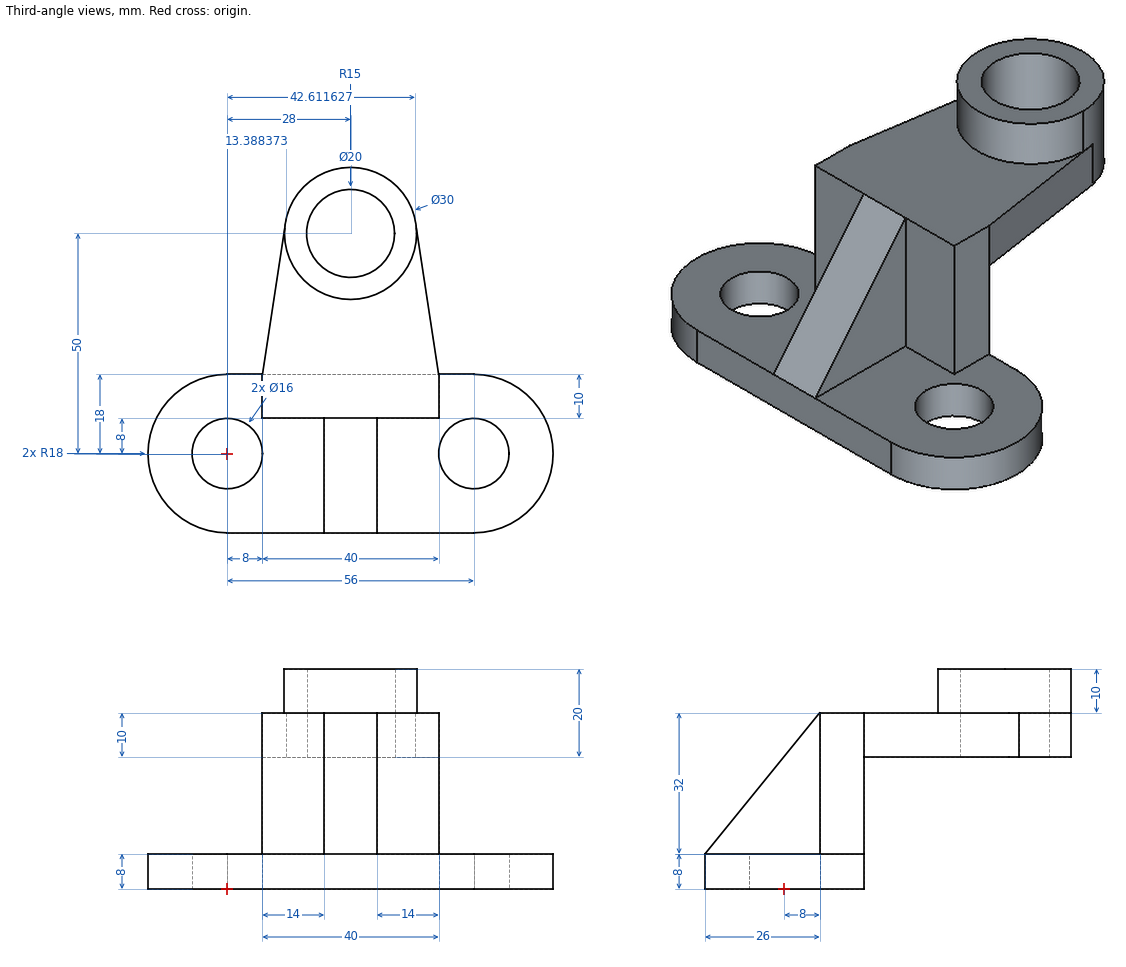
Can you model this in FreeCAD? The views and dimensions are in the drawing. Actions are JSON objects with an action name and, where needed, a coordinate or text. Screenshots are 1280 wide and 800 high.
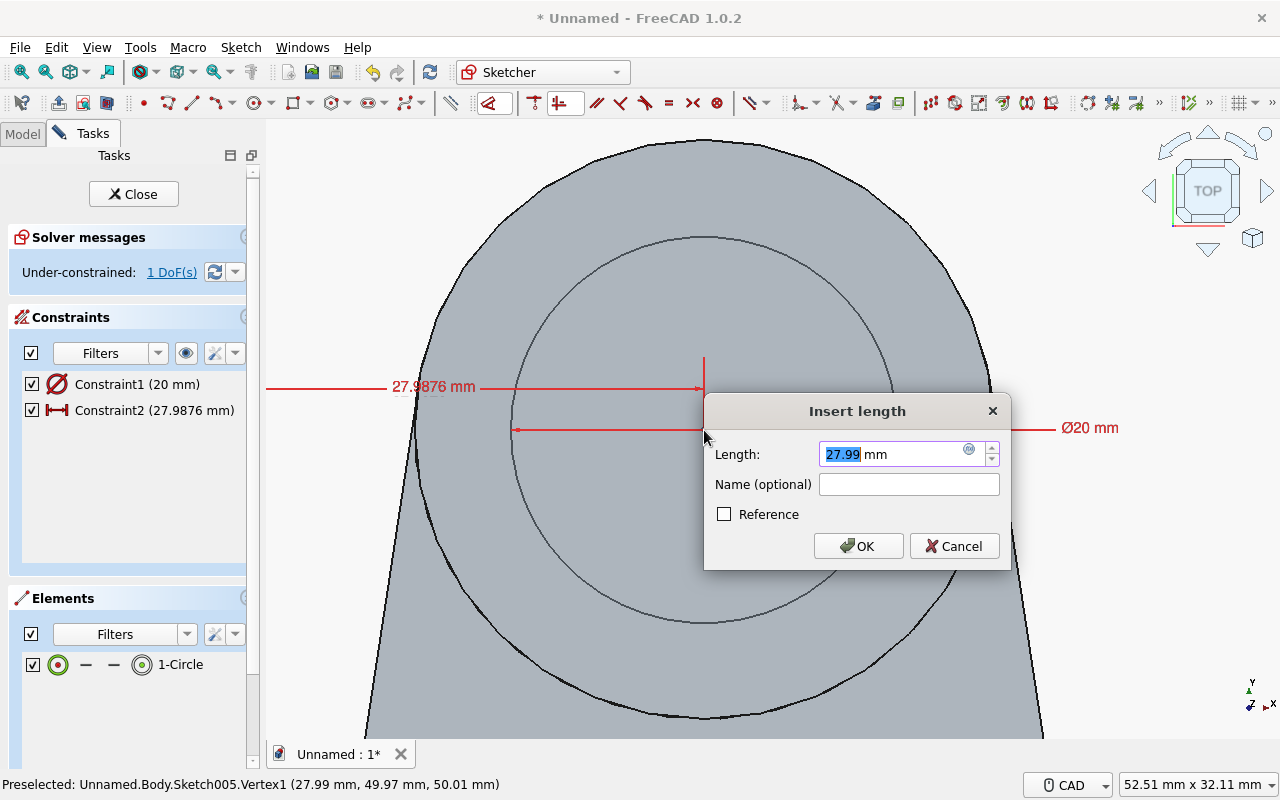
{"action": "type", "text": "28"}
{"action": "key", "text": "Return"}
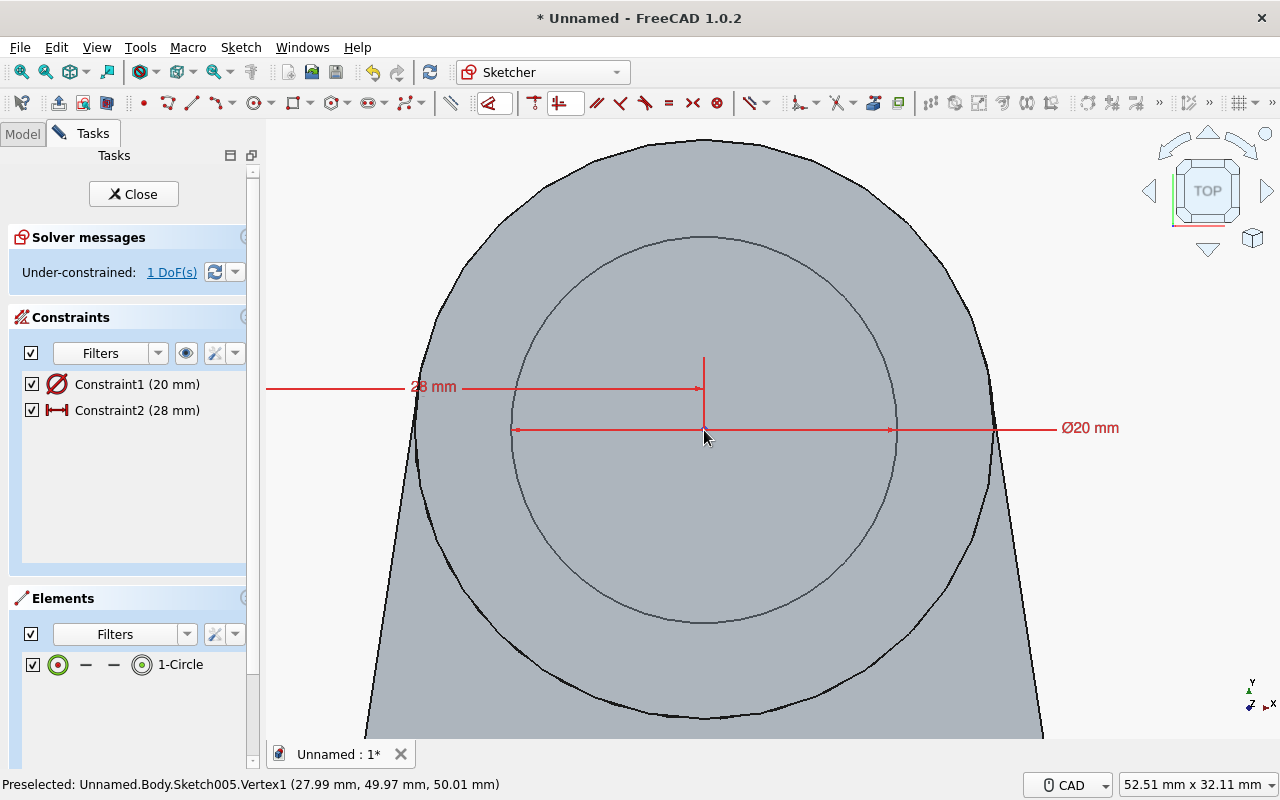
{"action": "left_click", "coordinate": [704, 430]}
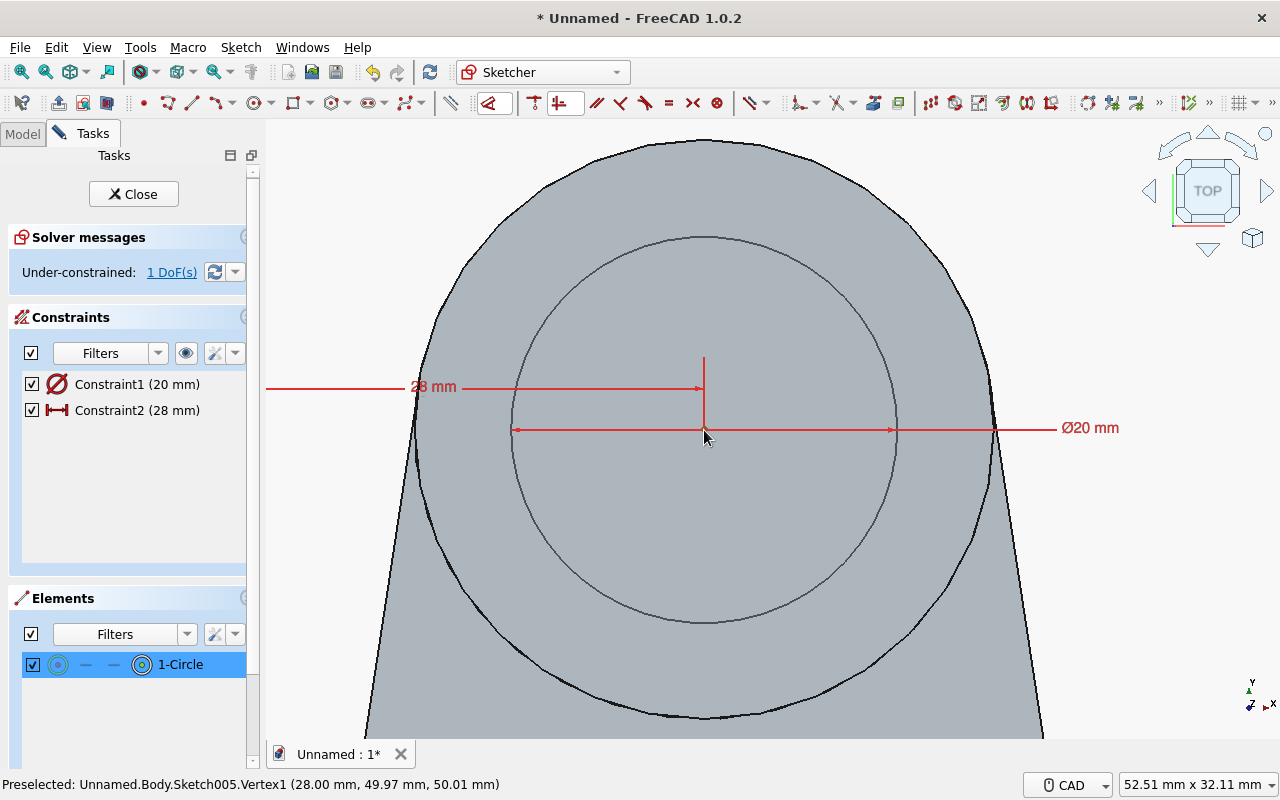
{"action": "key", "text": "i"}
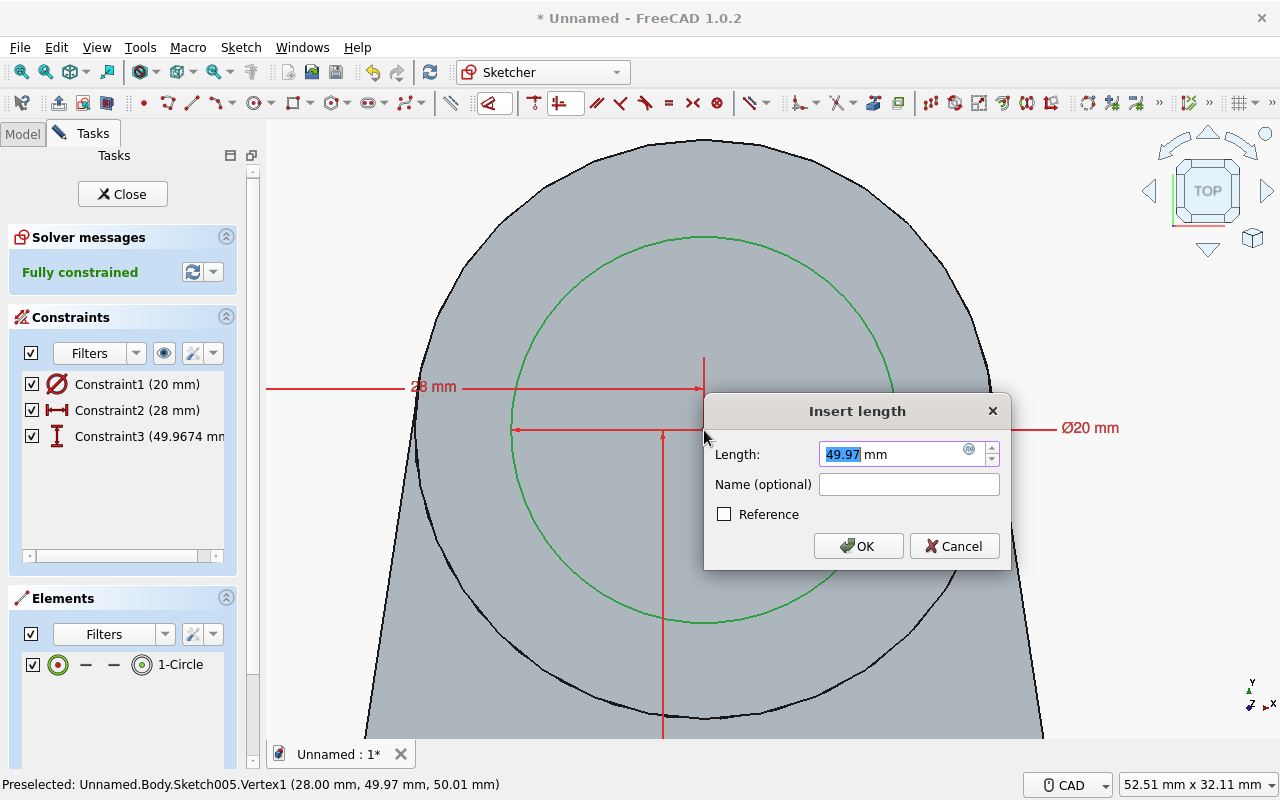
{"action": "type", "text": "50"}
{"action": "key", "text": "Return"}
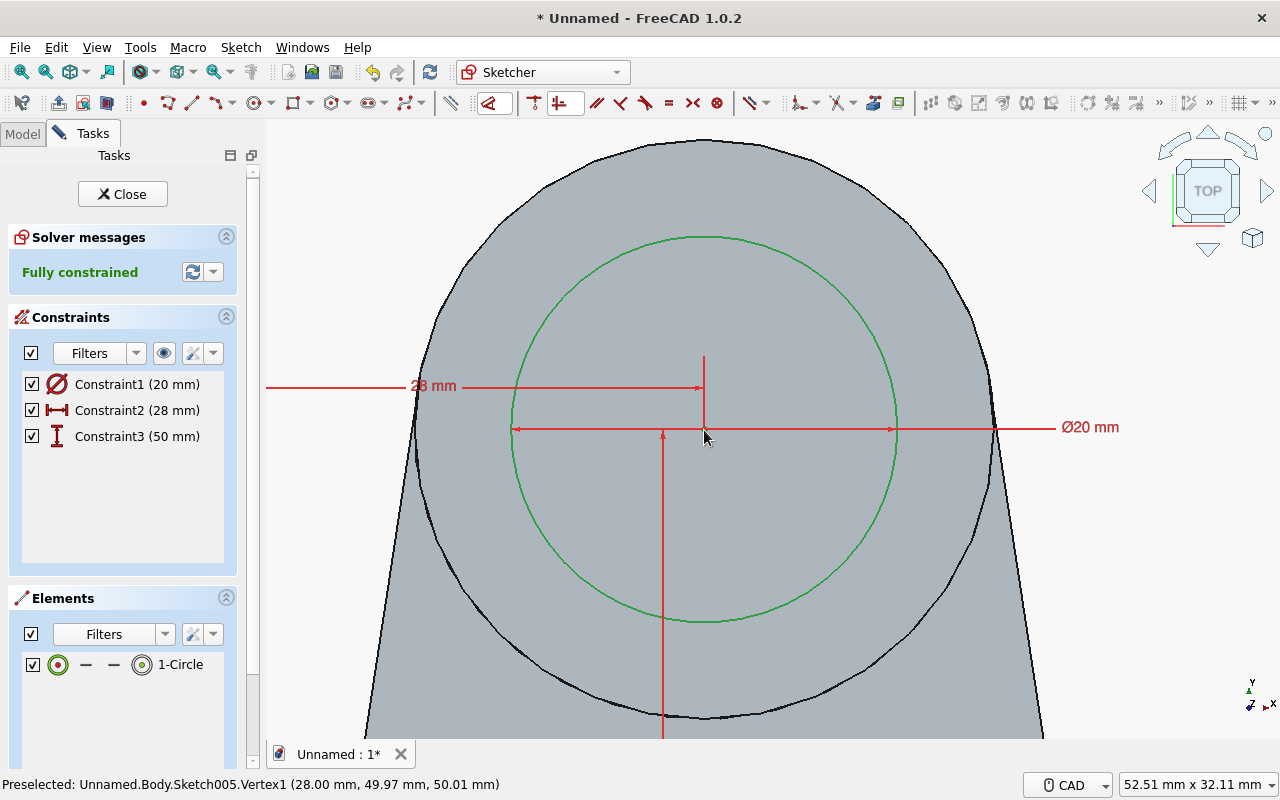
{"action": "left_click", "coordinate": [123, 194]}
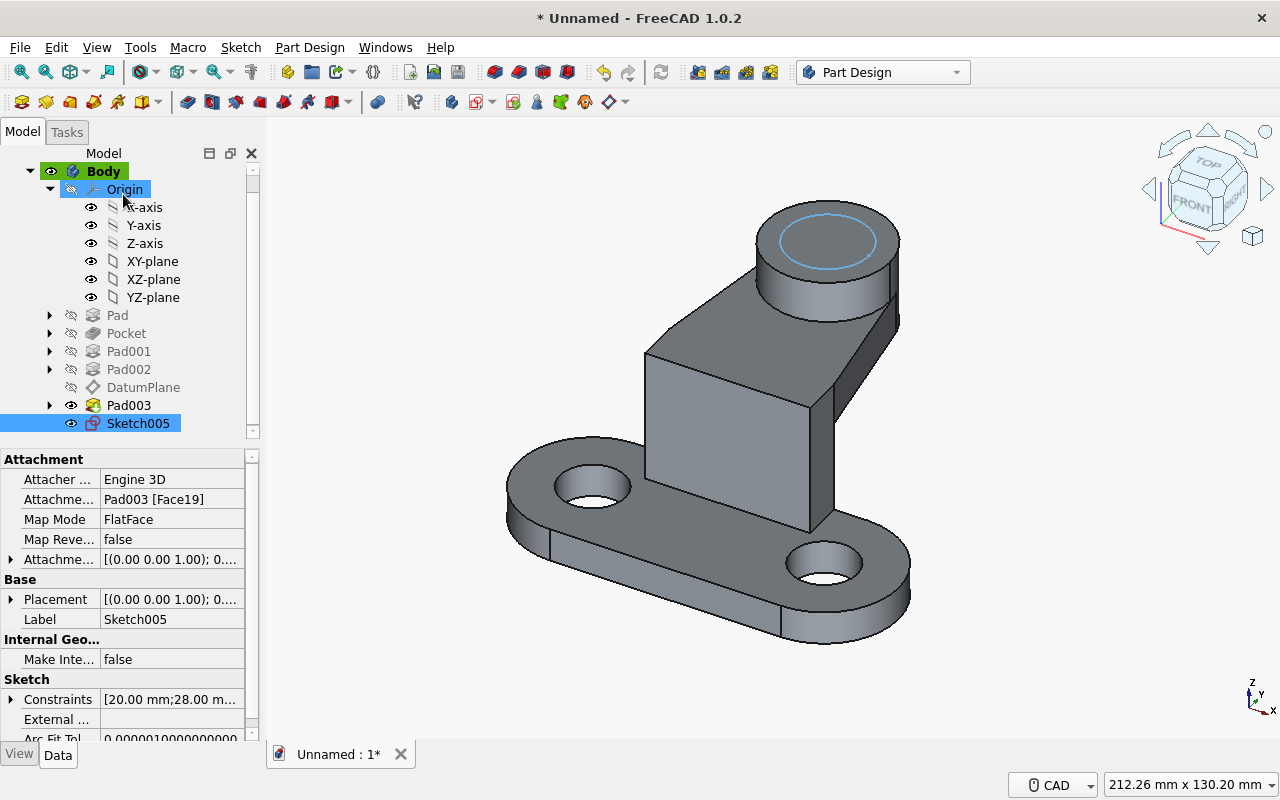
{"action": "left_click", "coordinate": [188, 102]}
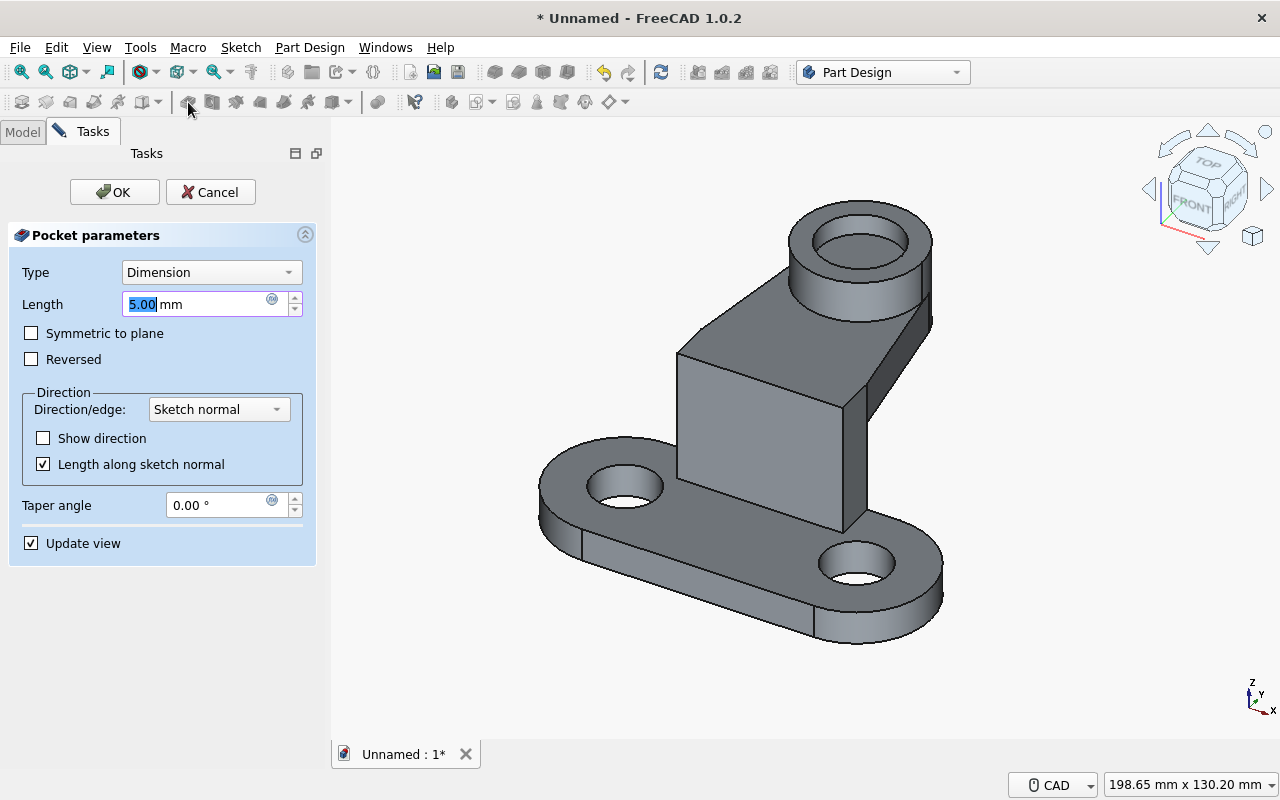
{"action": "type", "text": "20"}
{"action": "key", "text": "Tab"}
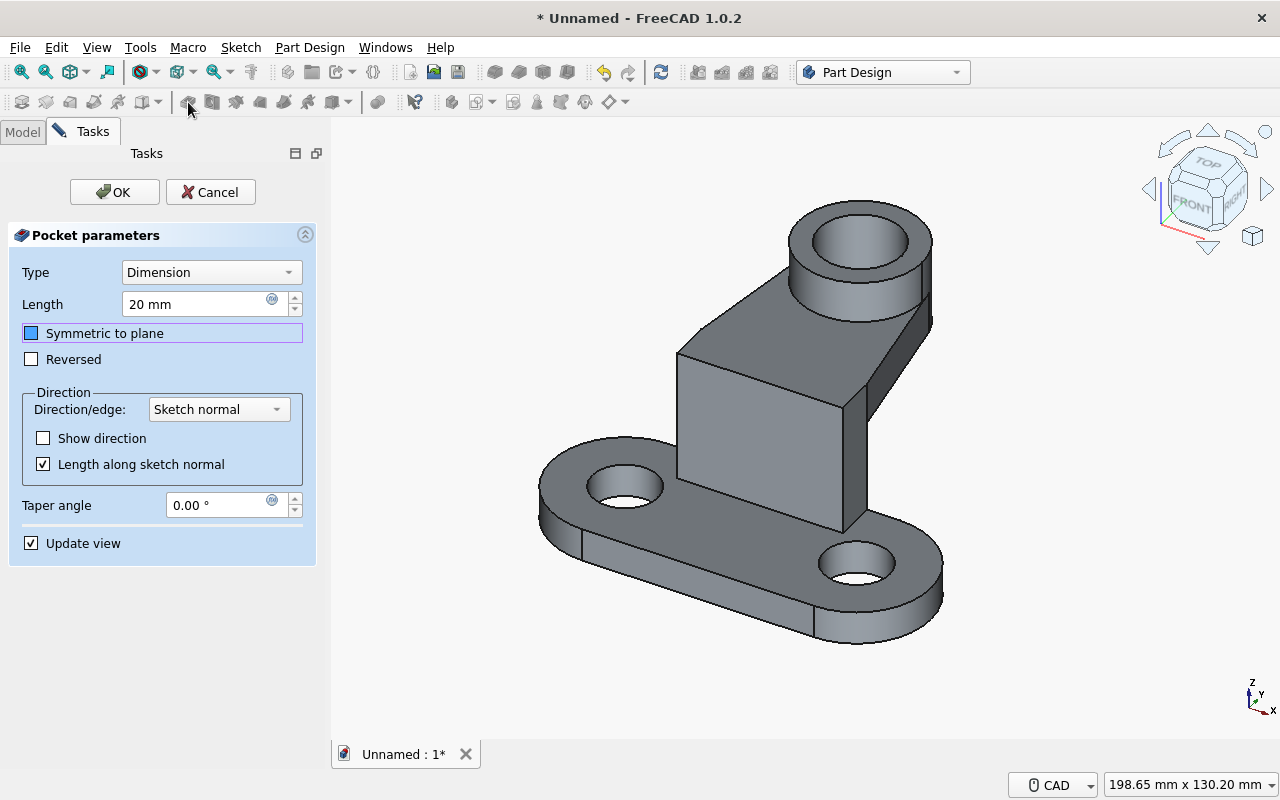
{"action": "left_click", "coordinate": [115, 192]}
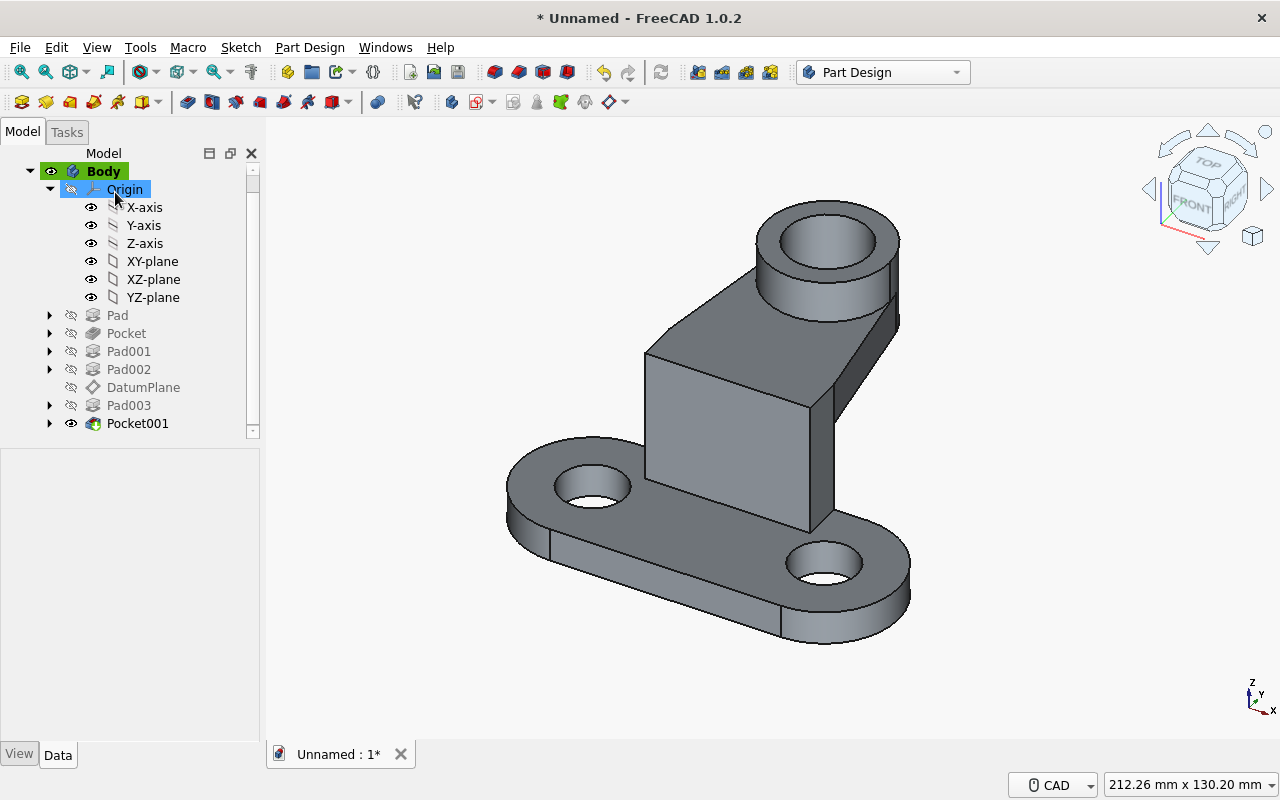
{"action": "left_click", "coordinate": [822, 422]}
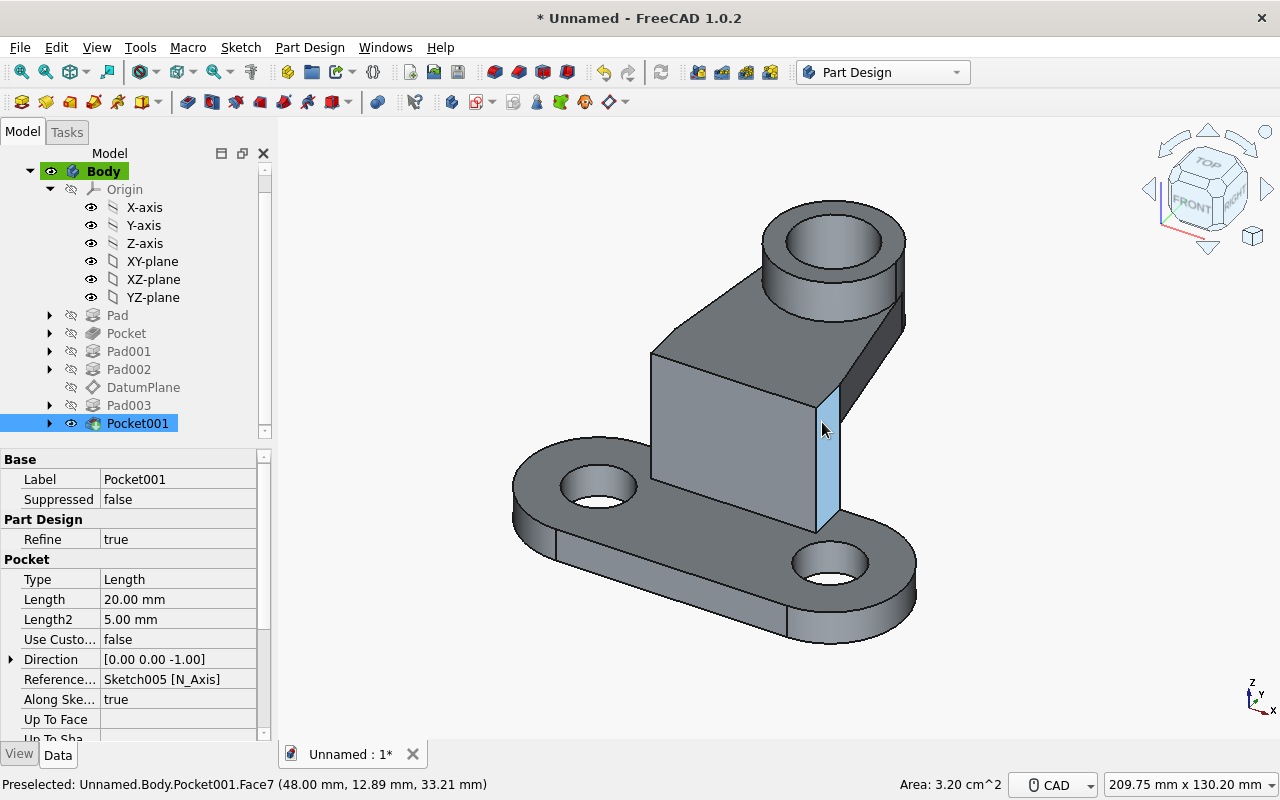
{"action": "left_click", "coordinate": [476, 102]}